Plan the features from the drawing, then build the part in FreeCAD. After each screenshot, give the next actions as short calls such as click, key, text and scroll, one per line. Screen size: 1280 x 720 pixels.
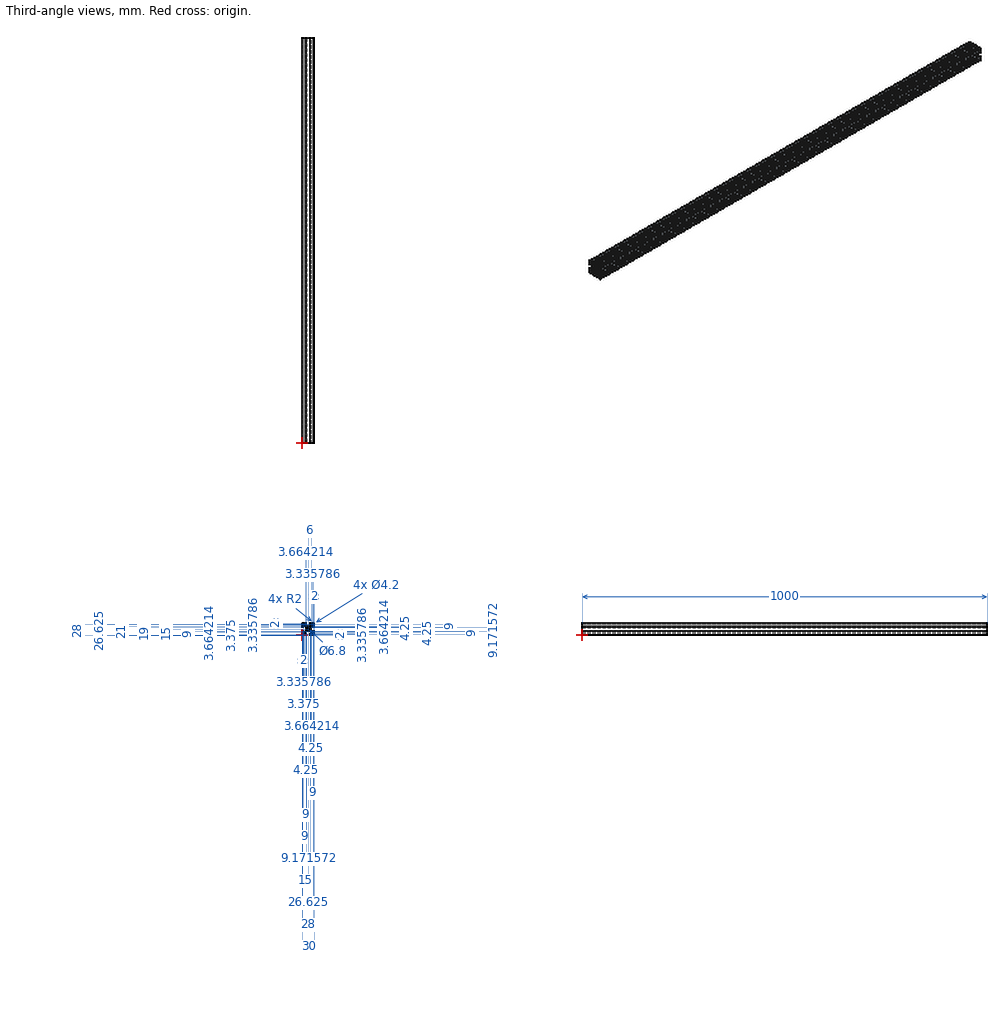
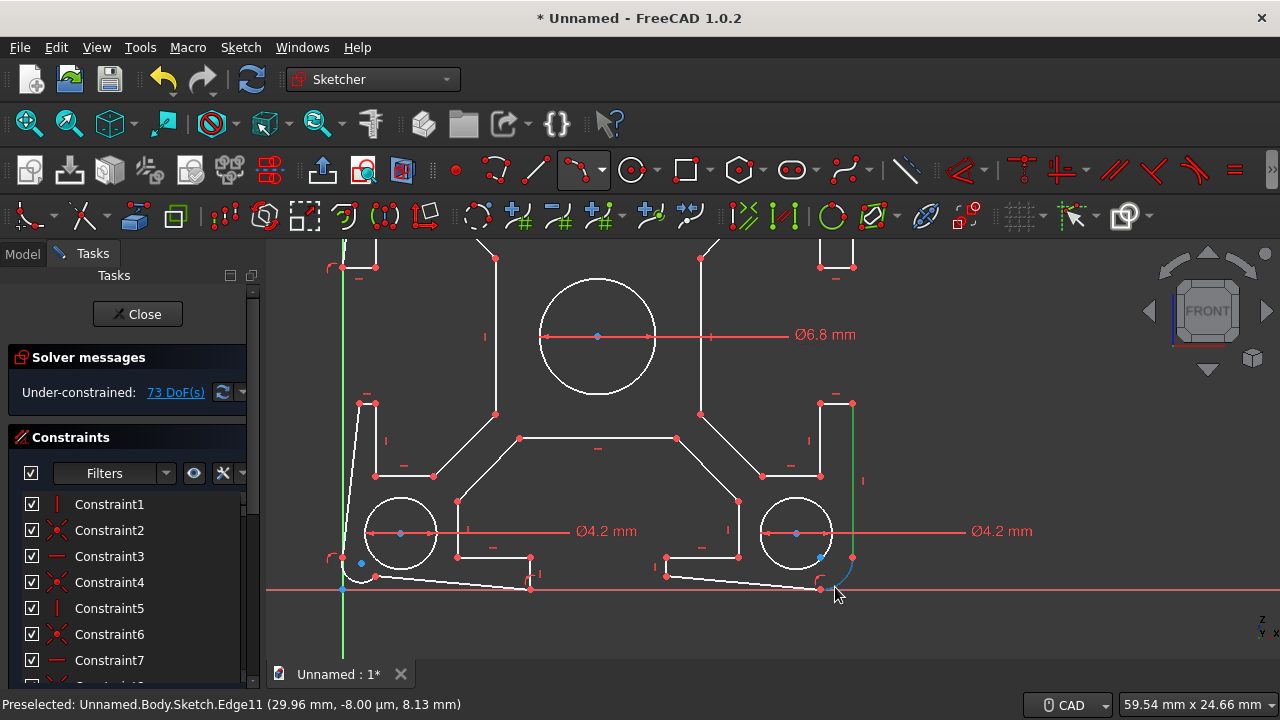
click(835, 586)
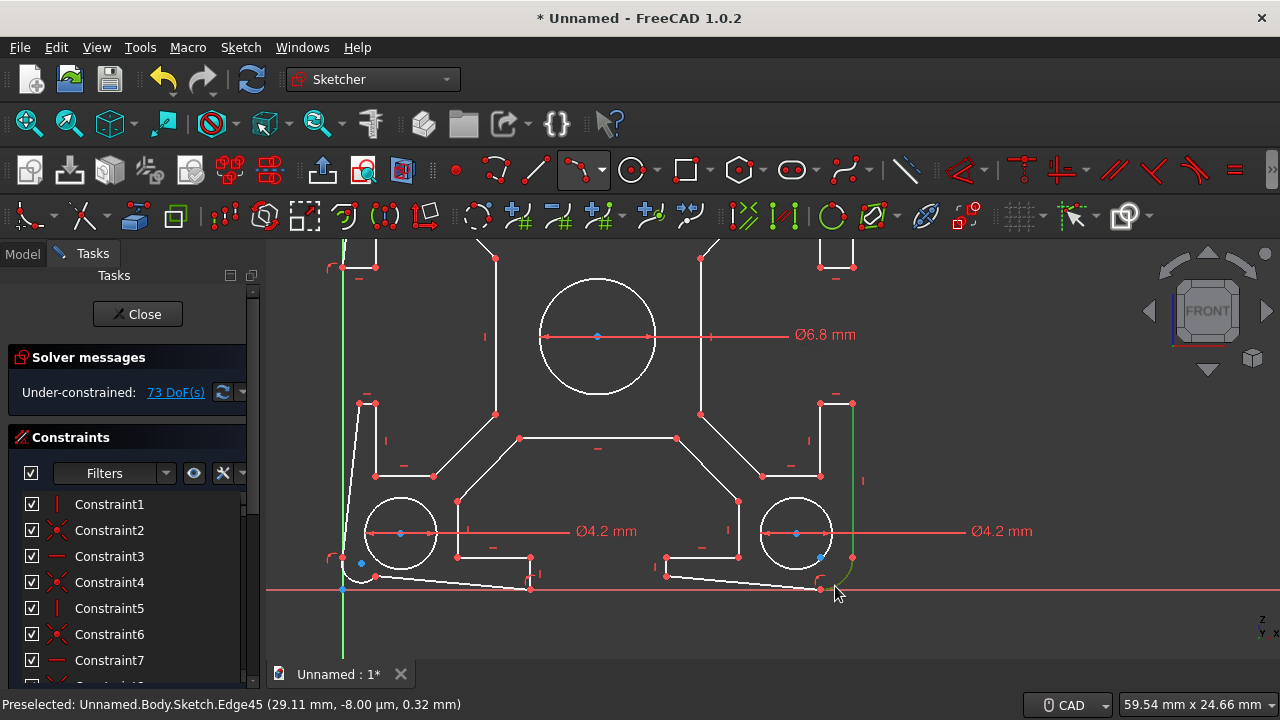
click(1196, 170)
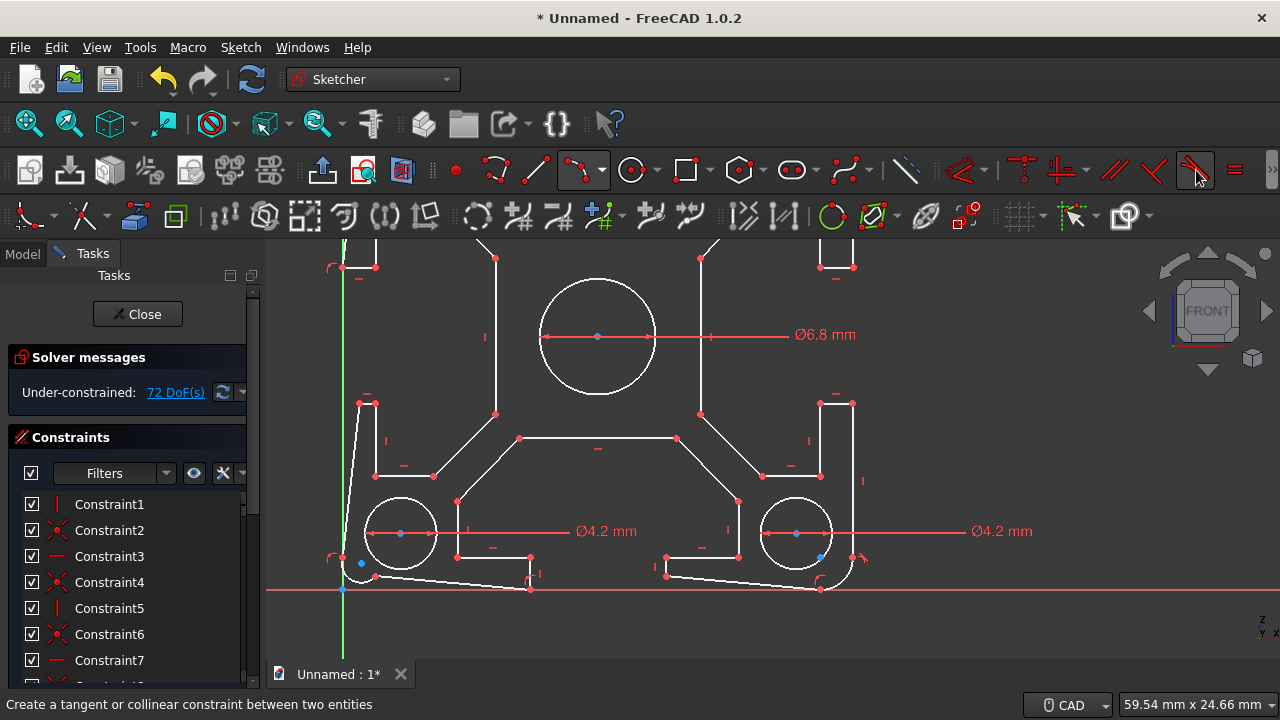
scroll(712, 580, up, 2)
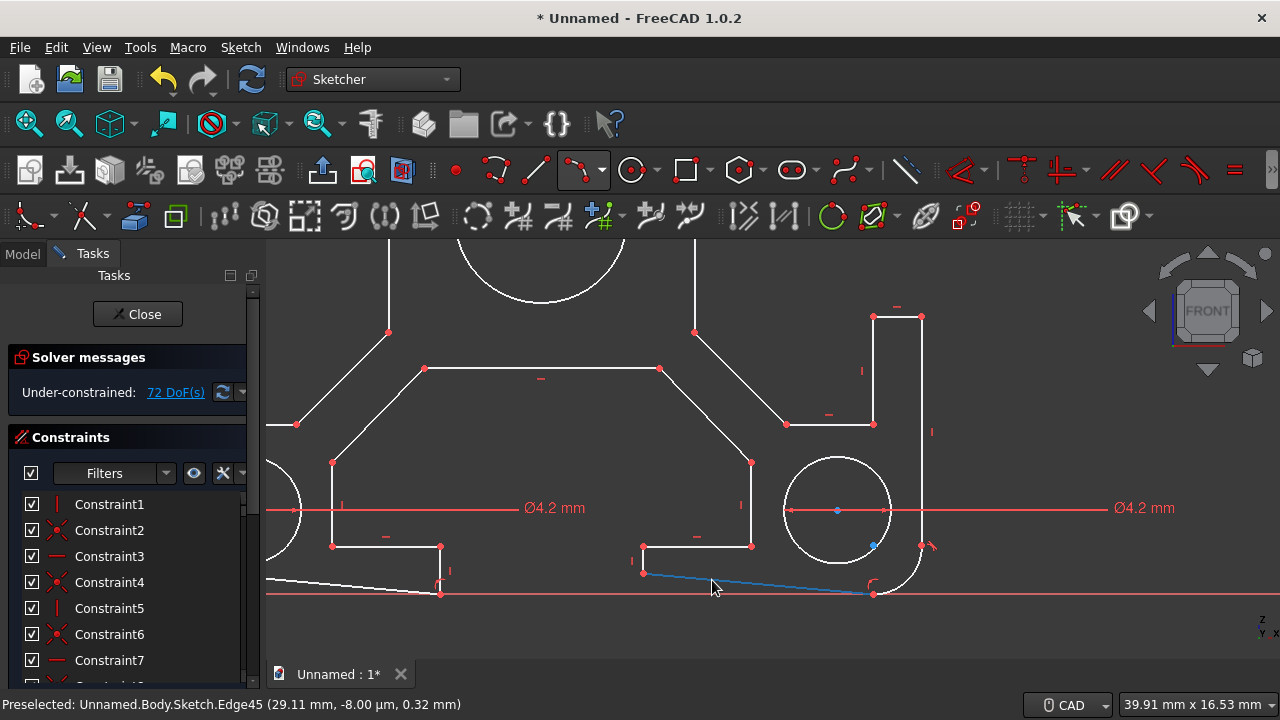
click(712, 580)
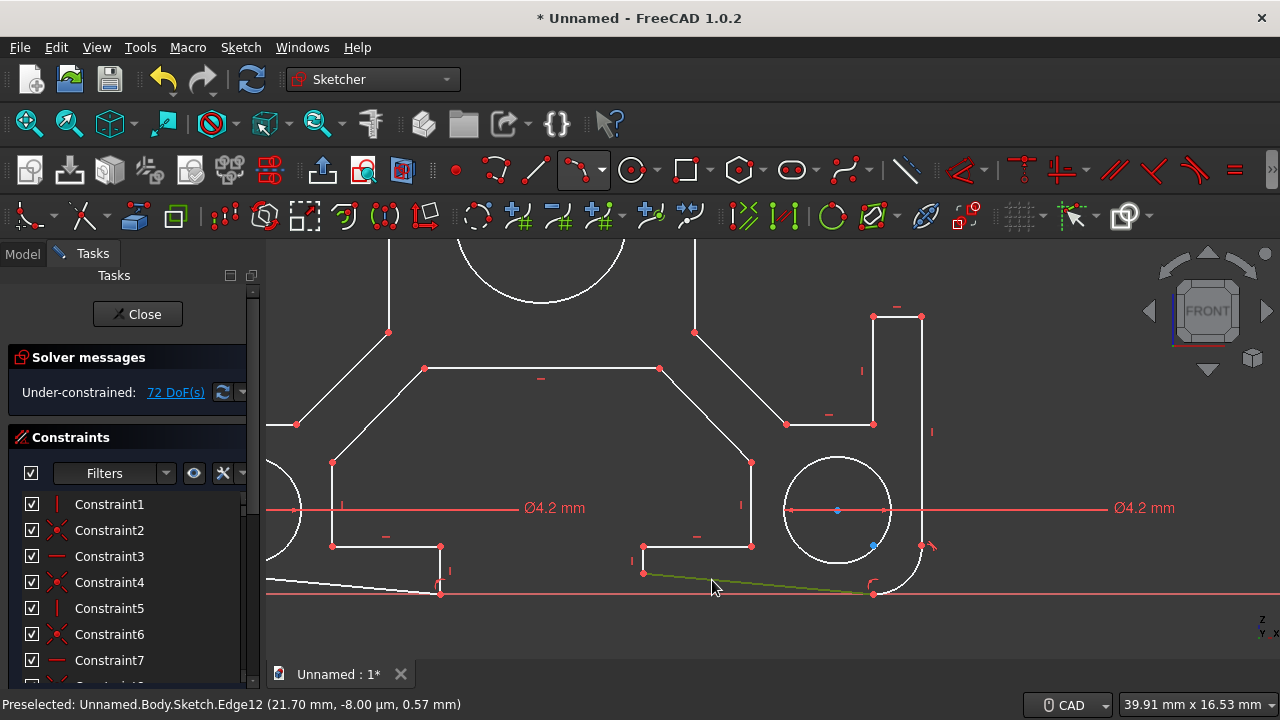
click(917, 568)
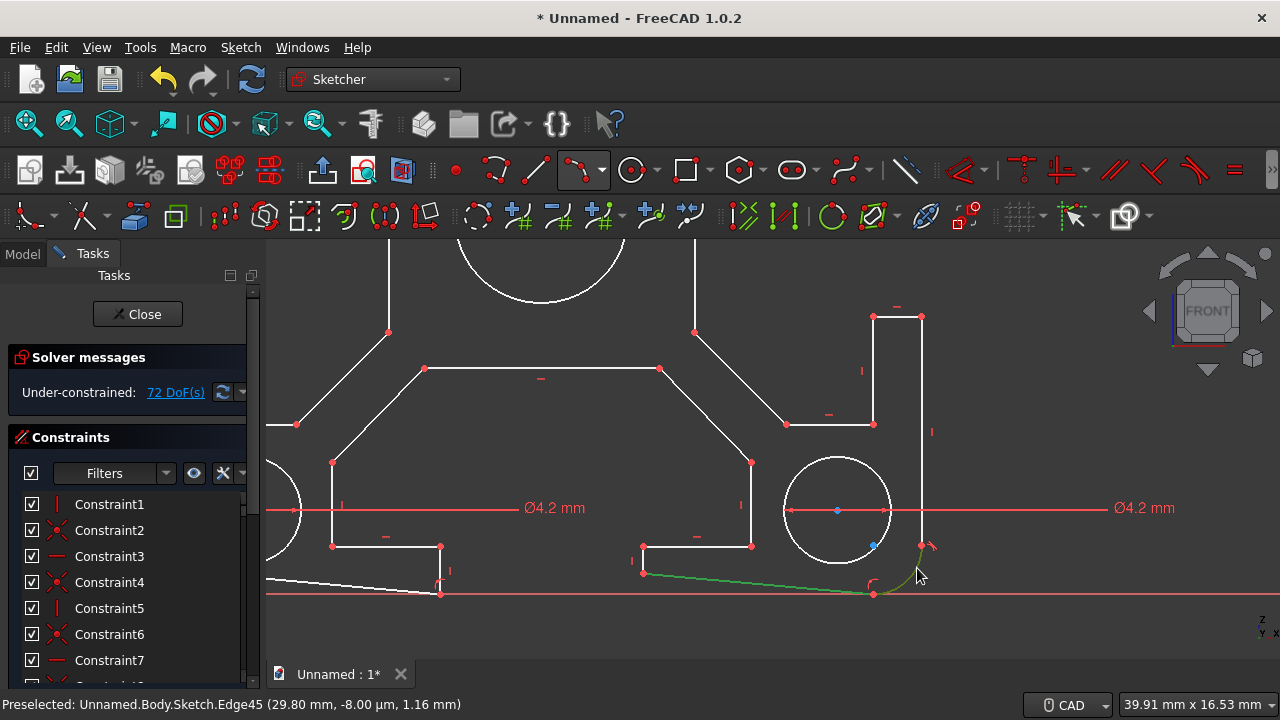
click(1196, 170)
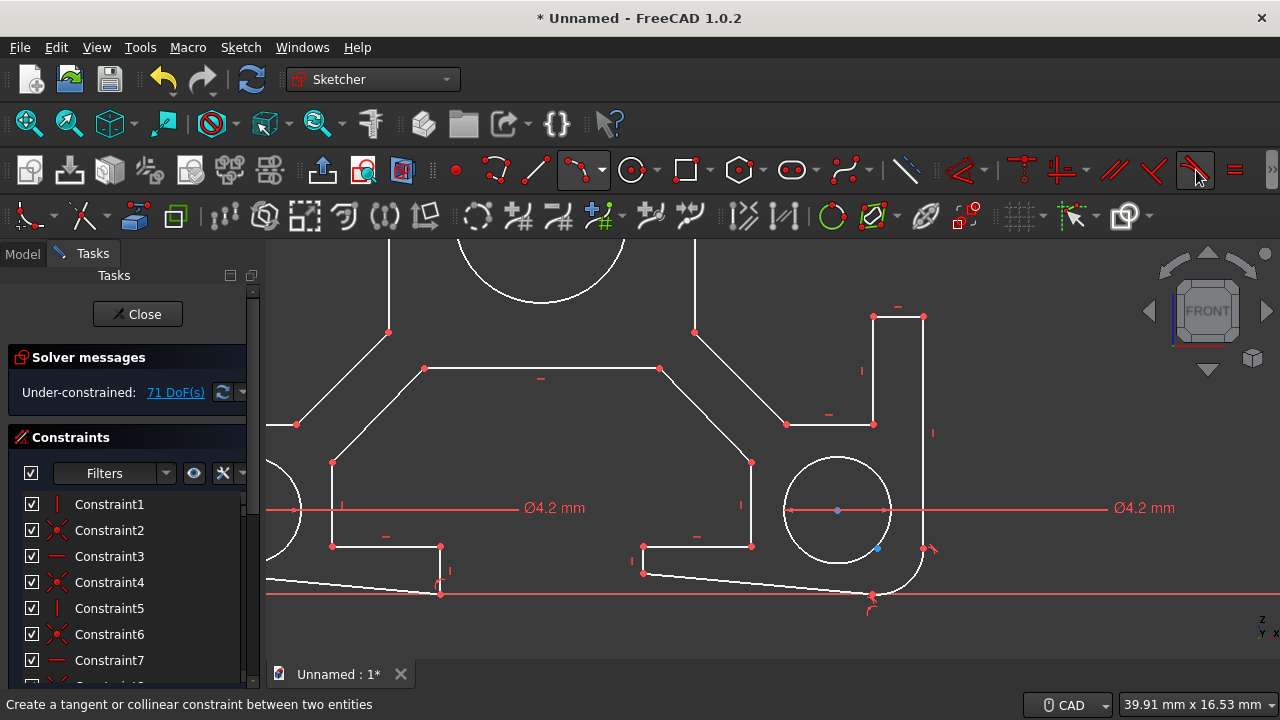
click(302, 582)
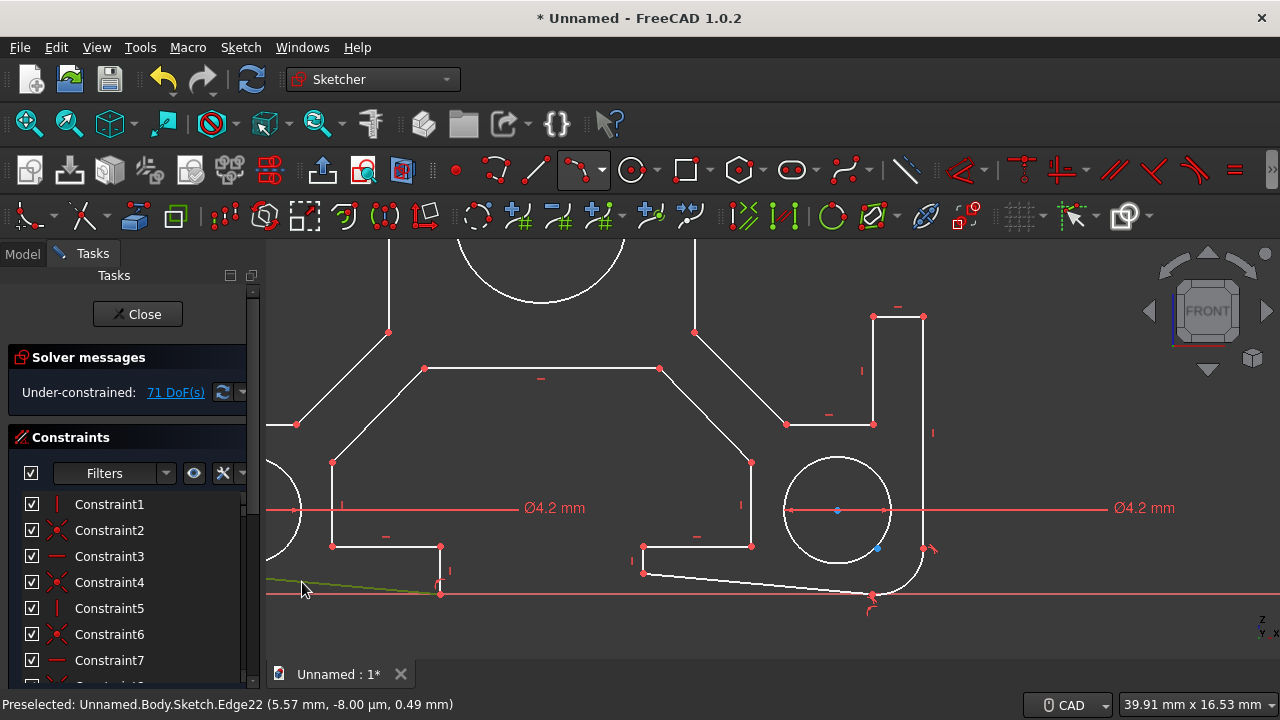
scroll(799, 586, down, 5)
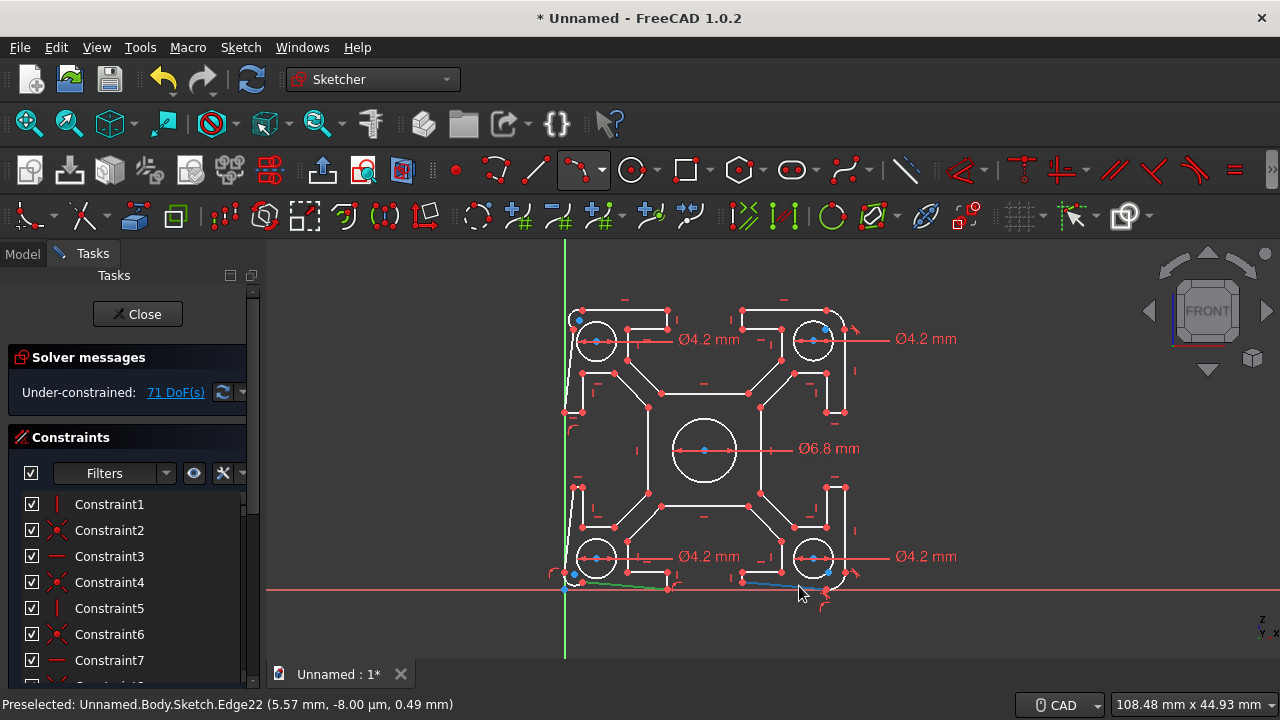
scroll(566, 580, up, 3)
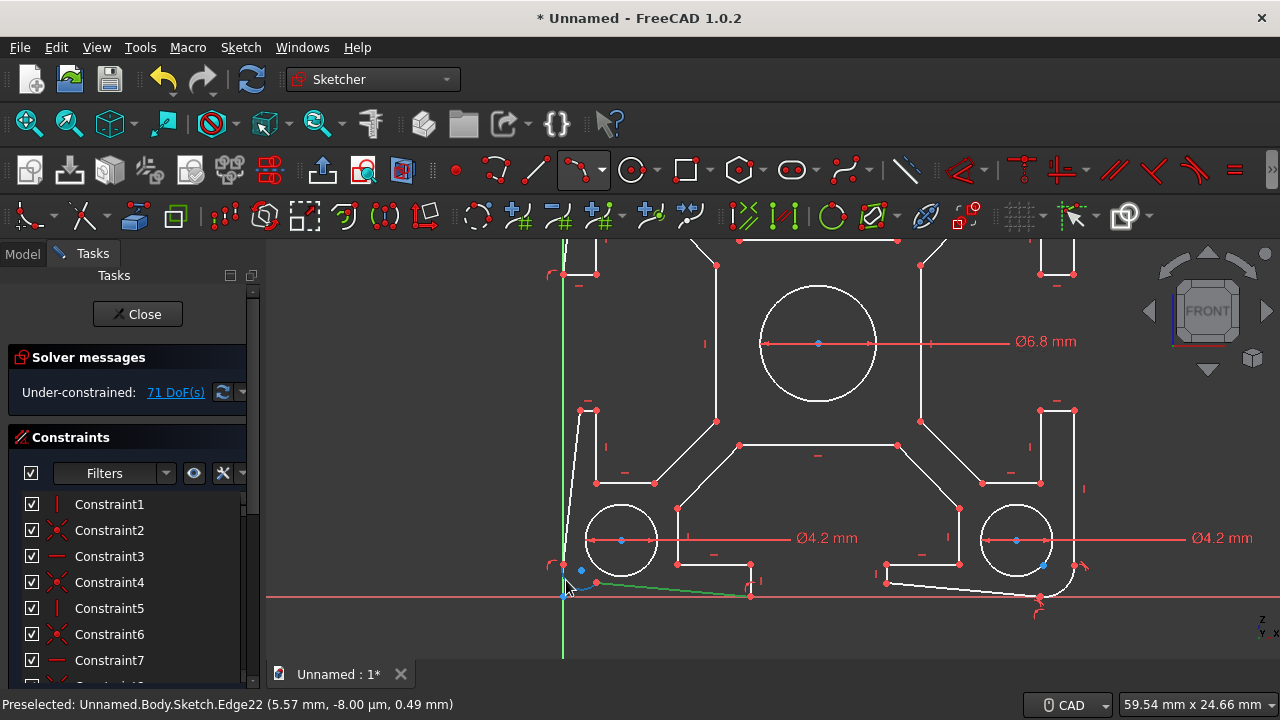
click(565, 580)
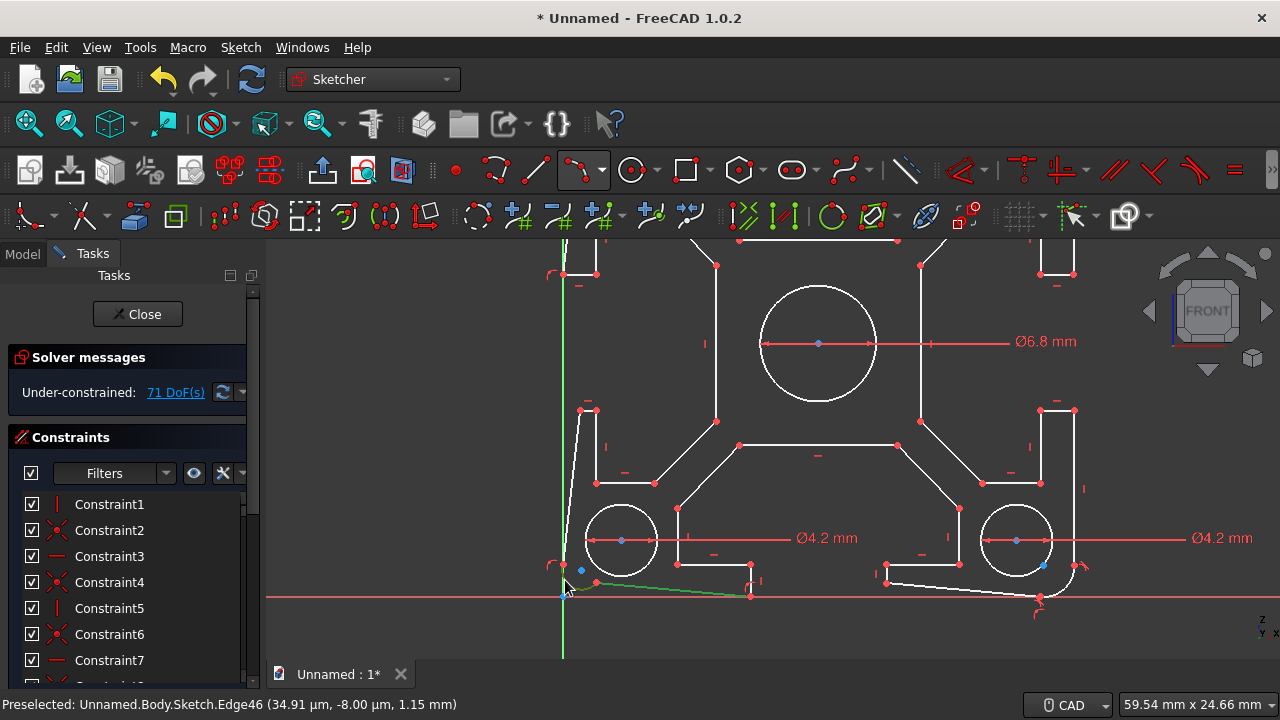
click(1196, 170)